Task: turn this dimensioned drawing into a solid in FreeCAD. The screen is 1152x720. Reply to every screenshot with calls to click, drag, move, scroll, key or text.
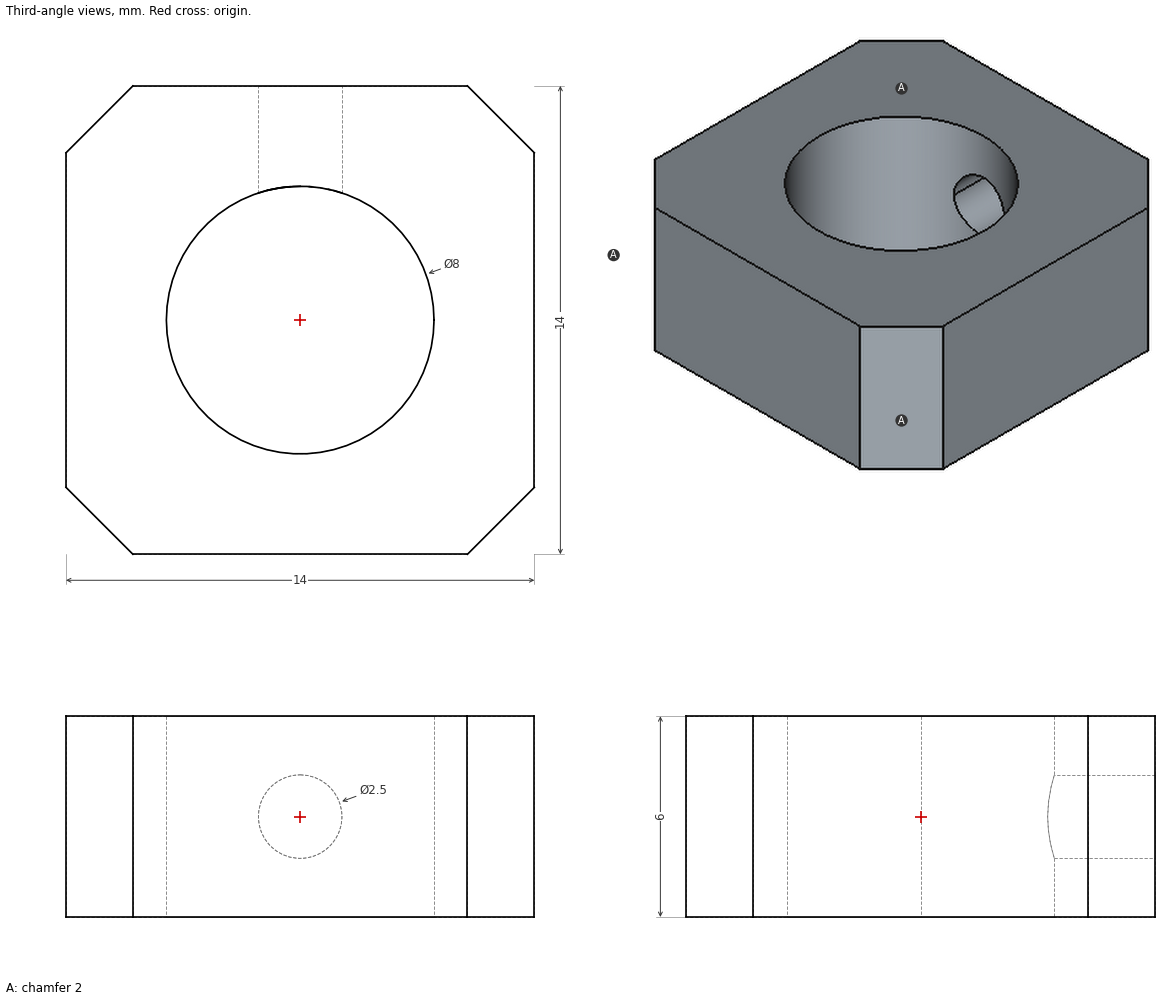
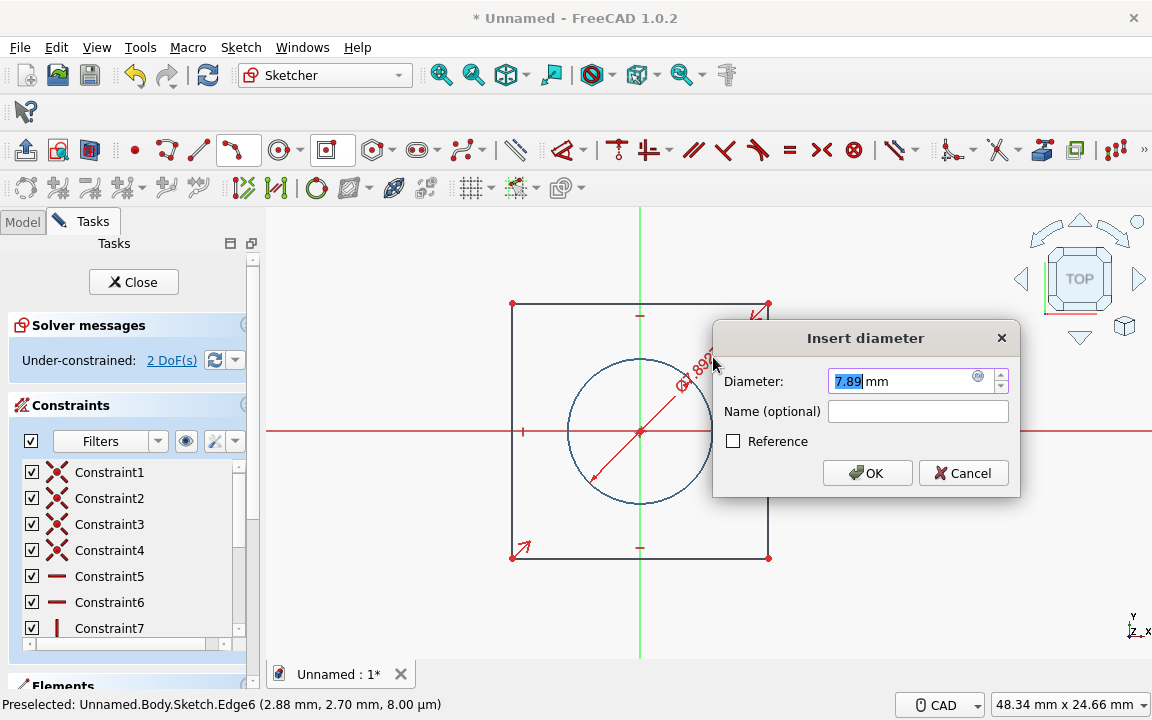
text(8)
key(Return)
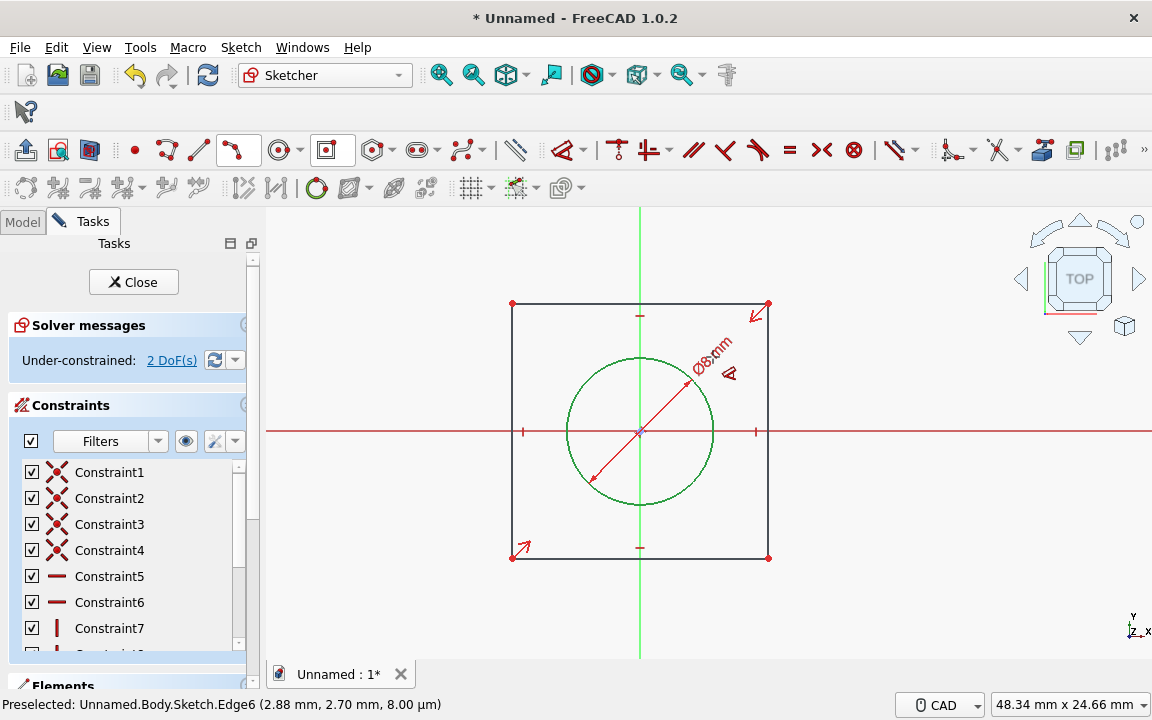
click(589, 559)
click(581, 593)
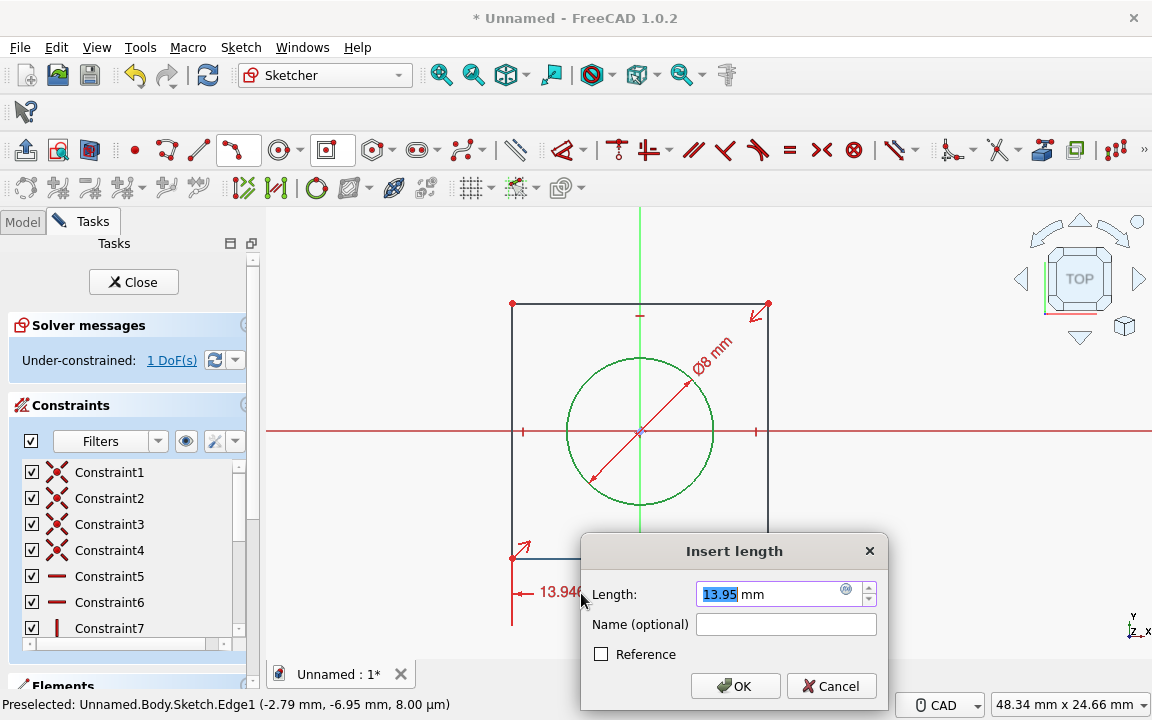
text(14)
key(Return)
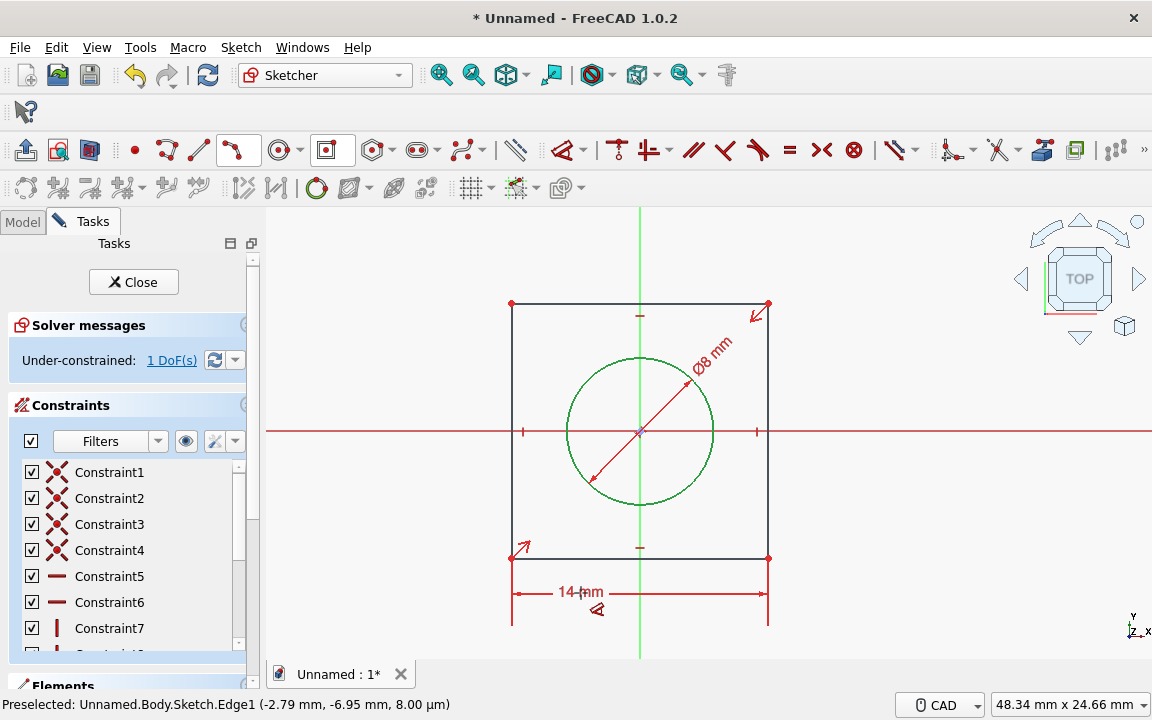
click(768, 482)
click(802, 373)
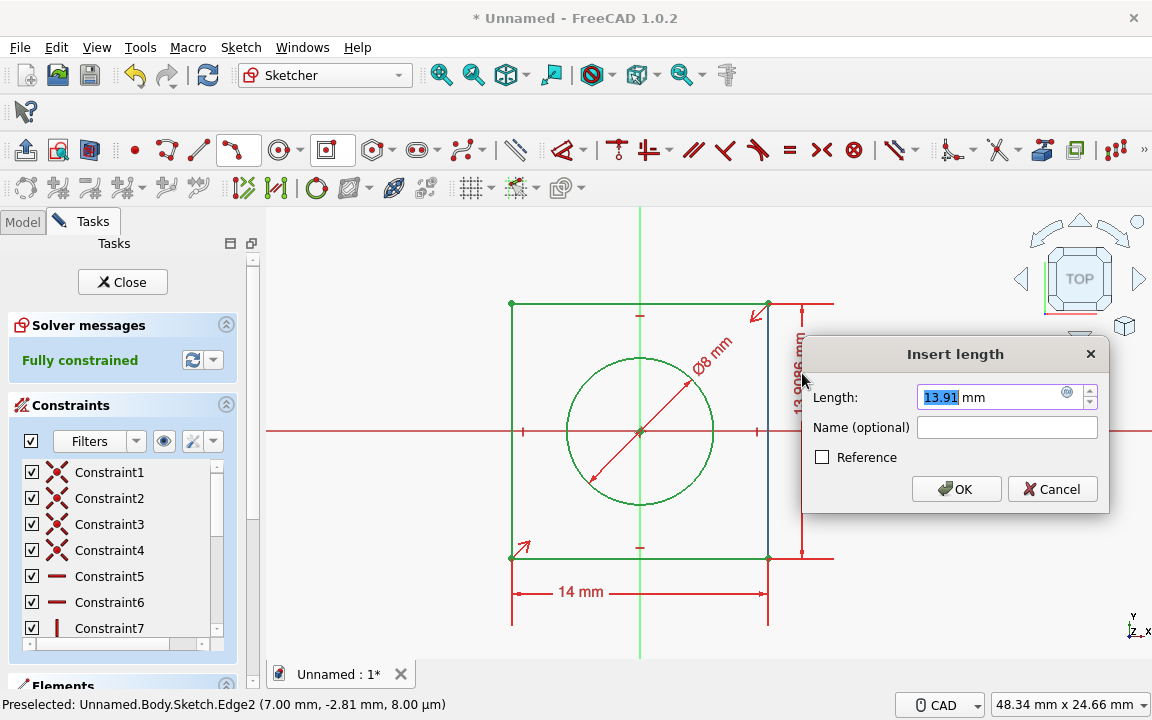
text(14)
key(Return)
key(Escape)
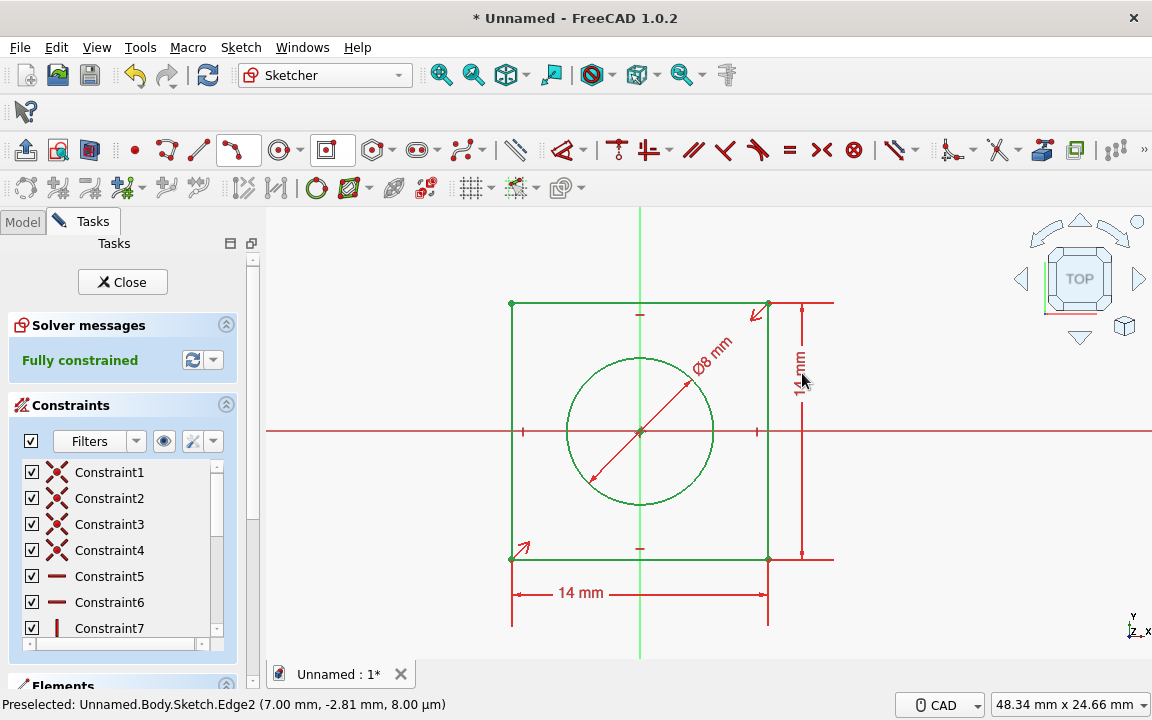
click(123, 282)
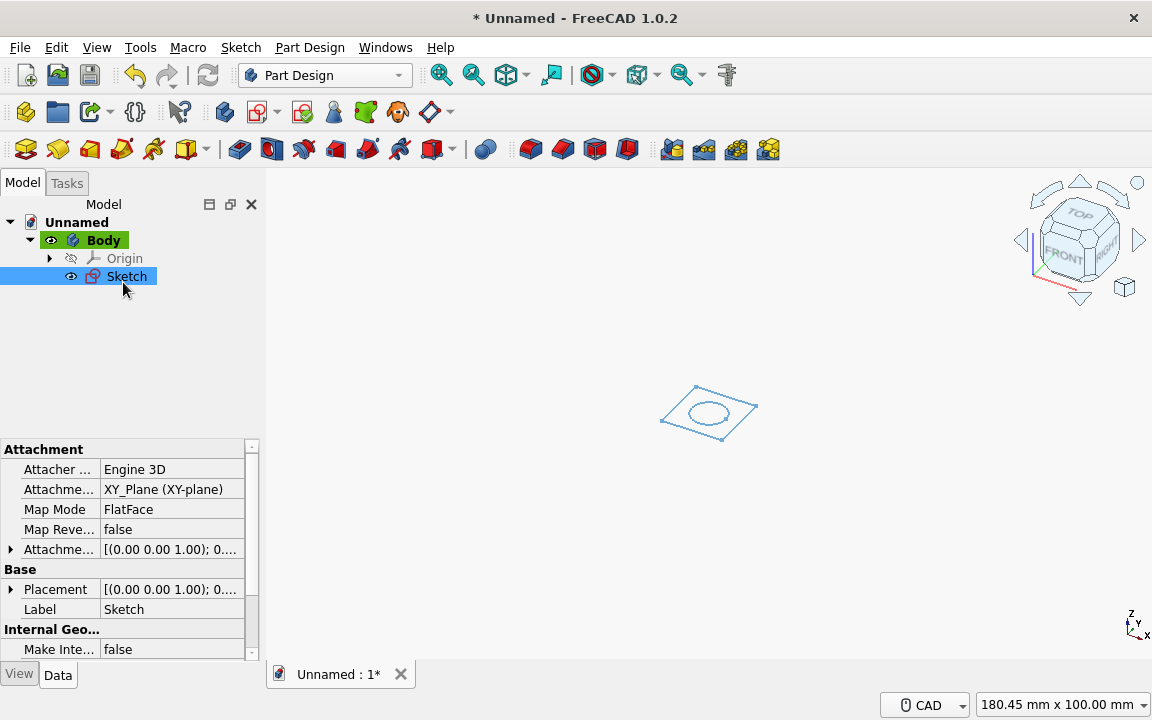
click(26, 150)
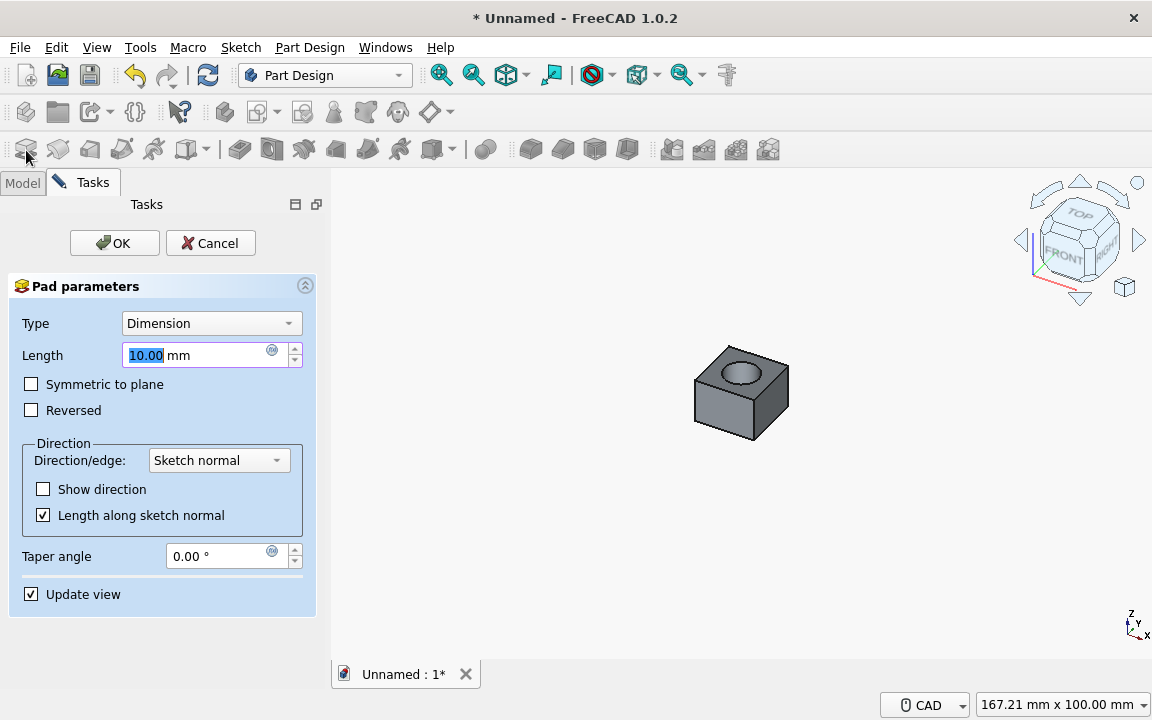
text(6)
key(Tab)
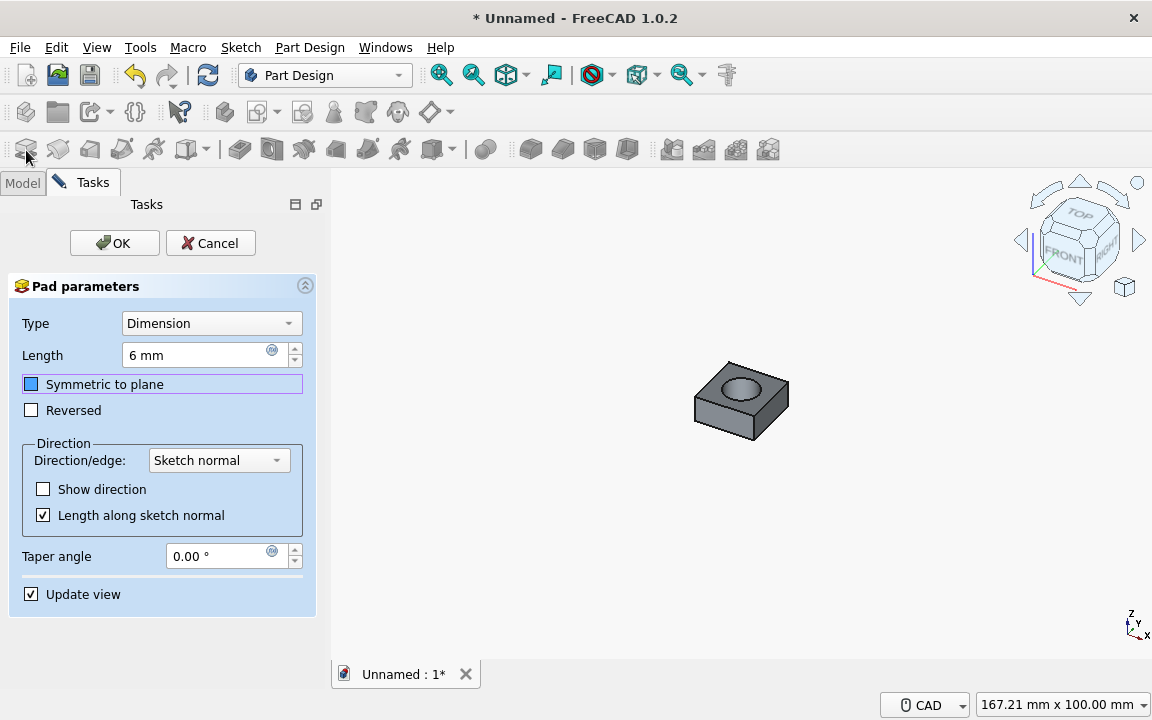
click(30, 384)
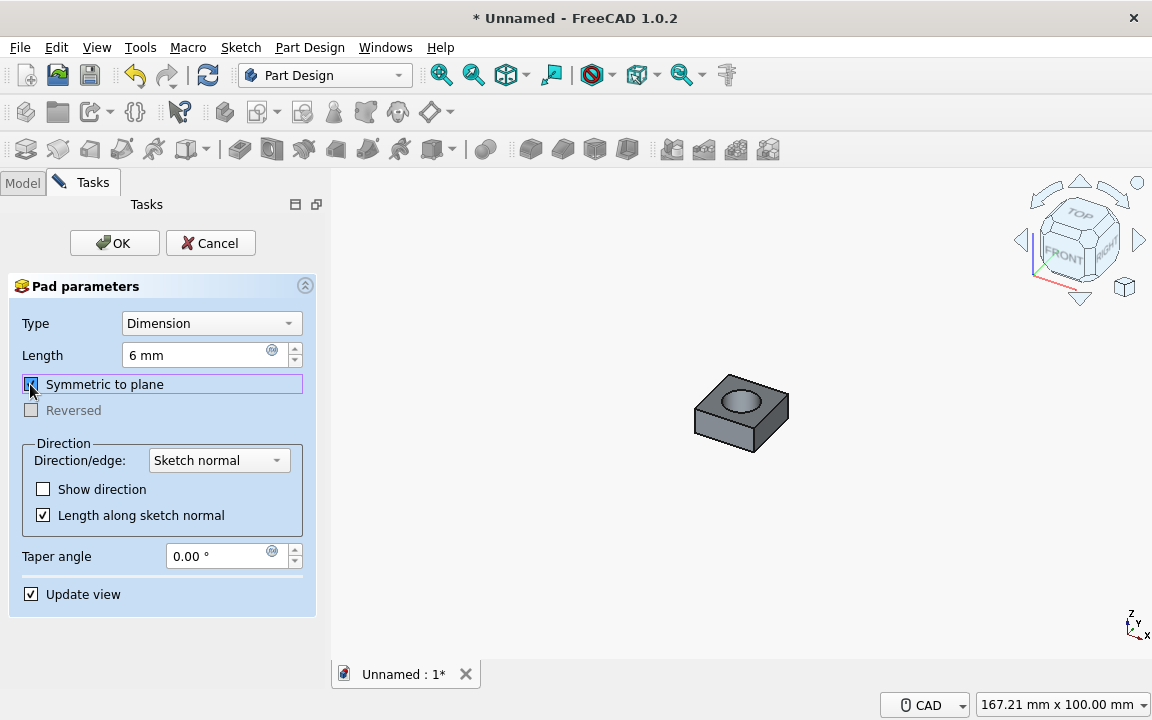
click(115, 243)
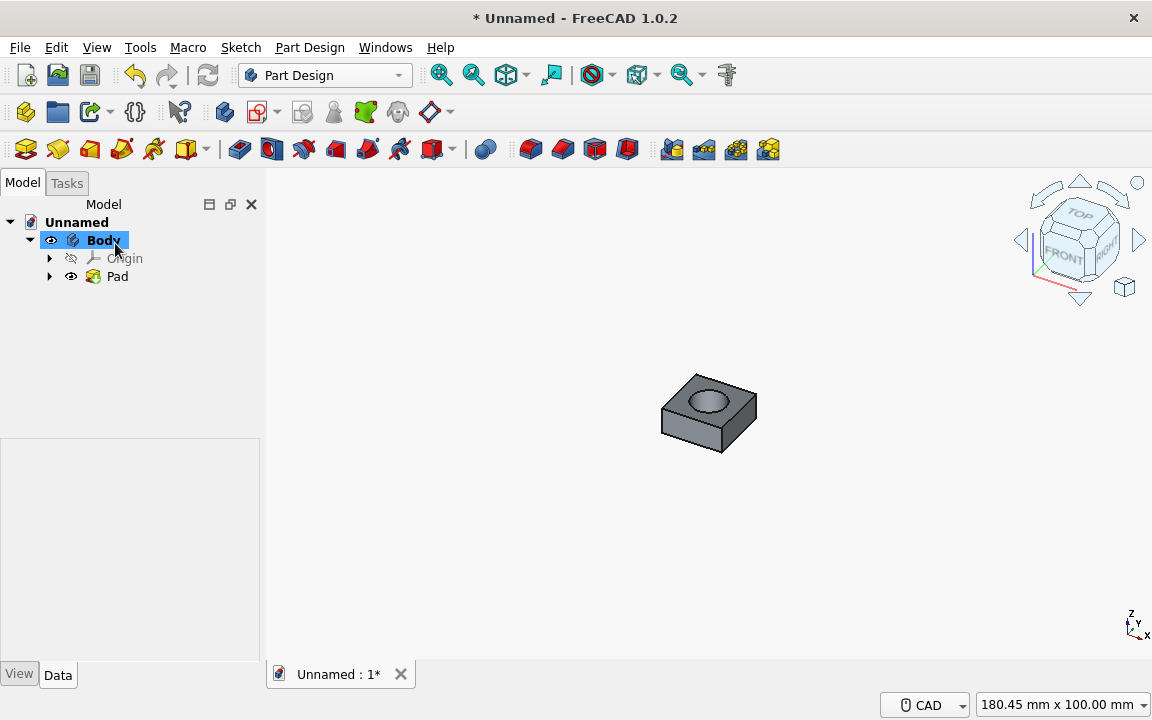
click(442, 76)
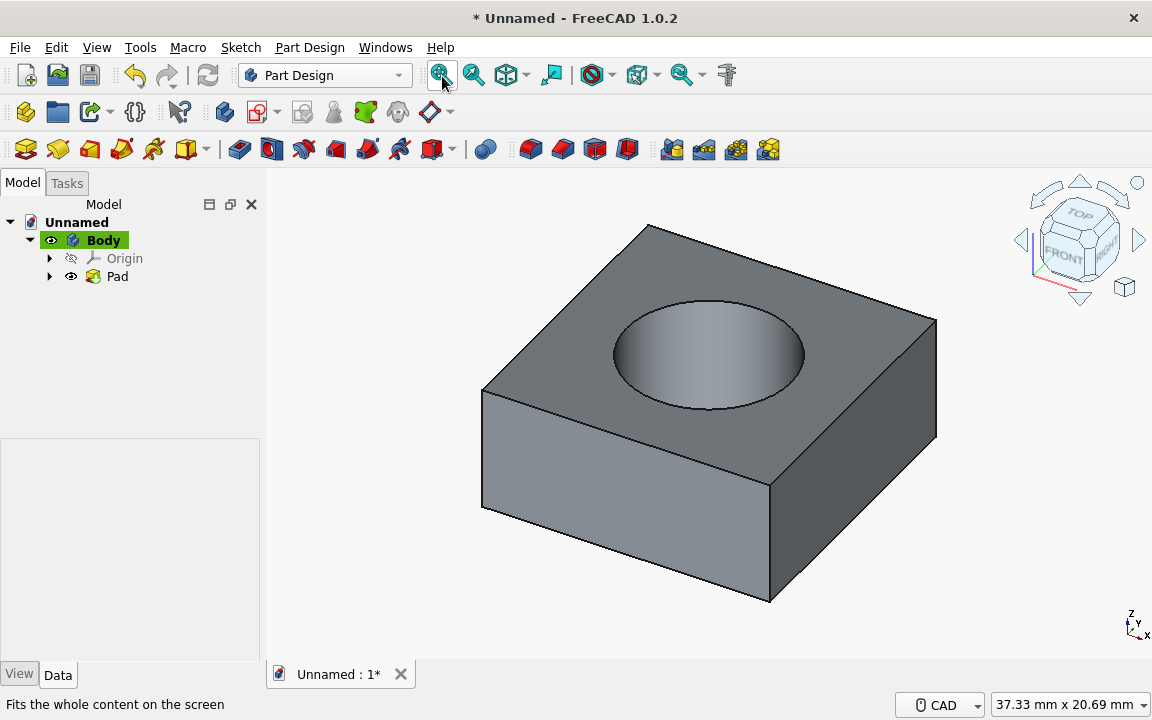
key(4)